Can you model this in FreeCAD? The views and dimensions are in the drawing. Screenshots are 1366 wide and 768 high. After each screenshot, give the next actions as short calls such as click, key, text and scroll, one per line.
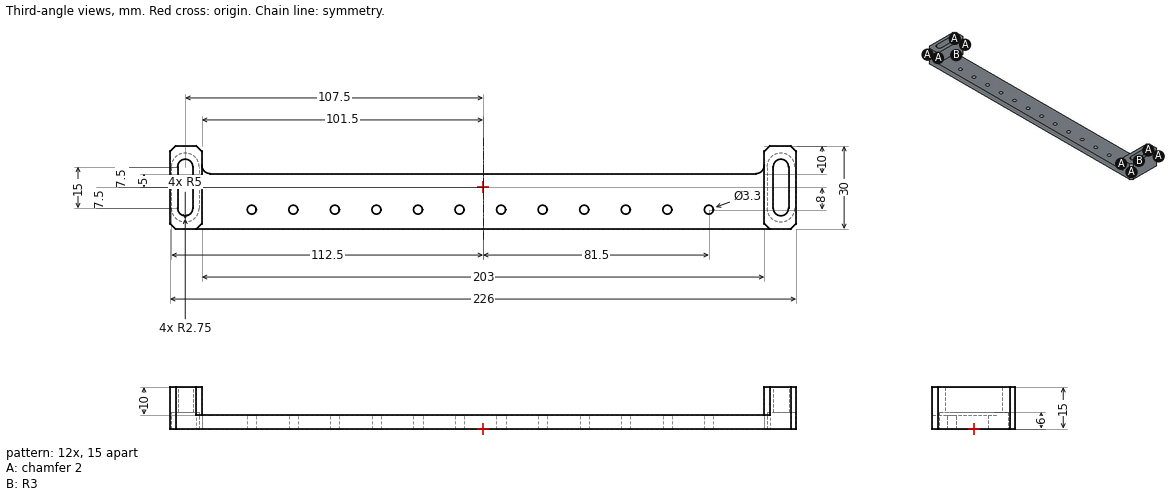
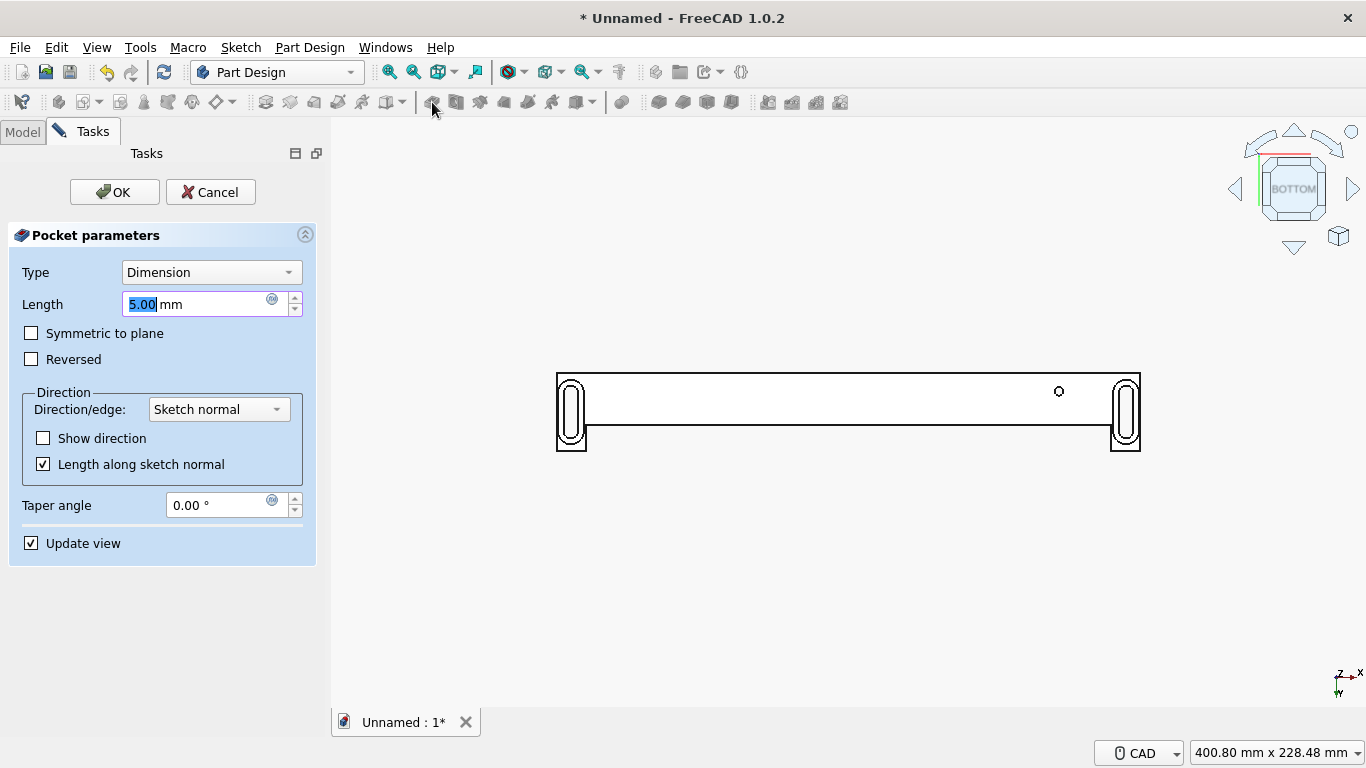
click(212, 272)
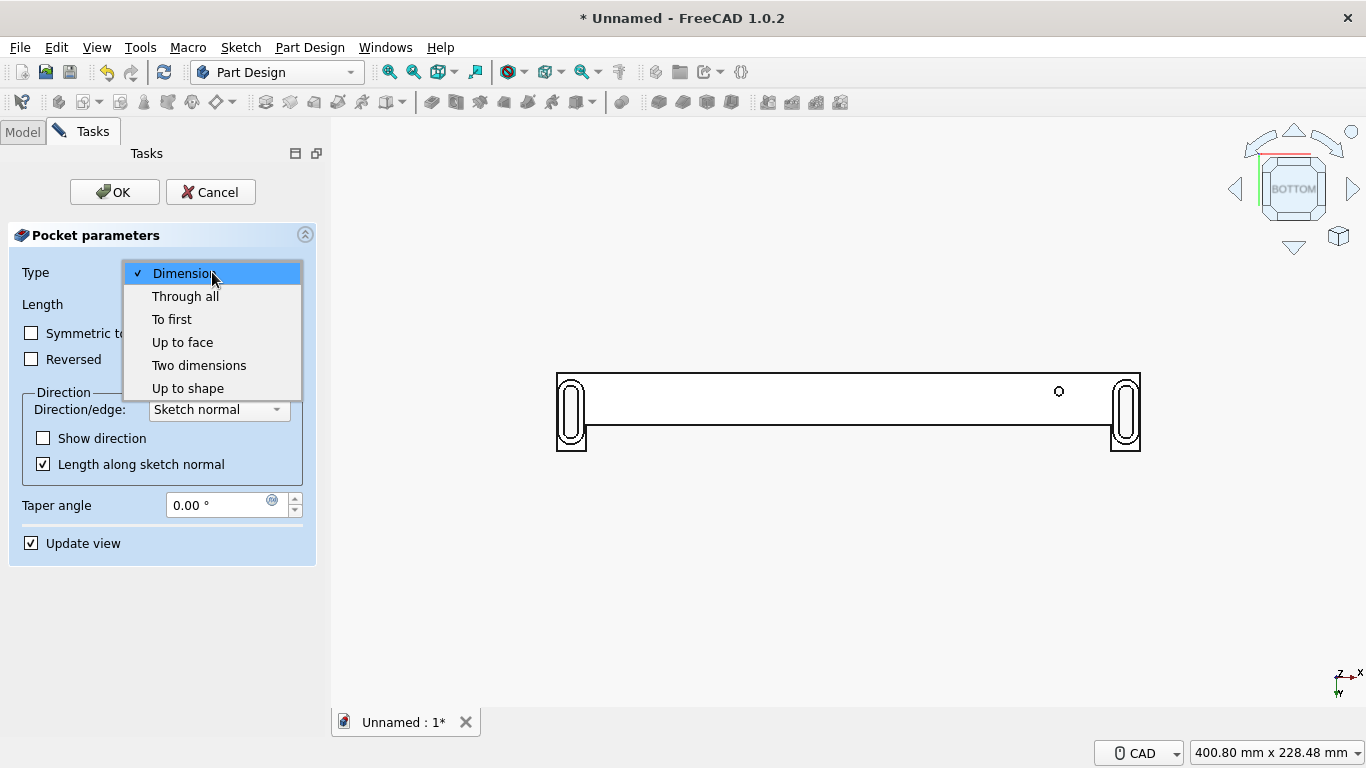
click(212, 296)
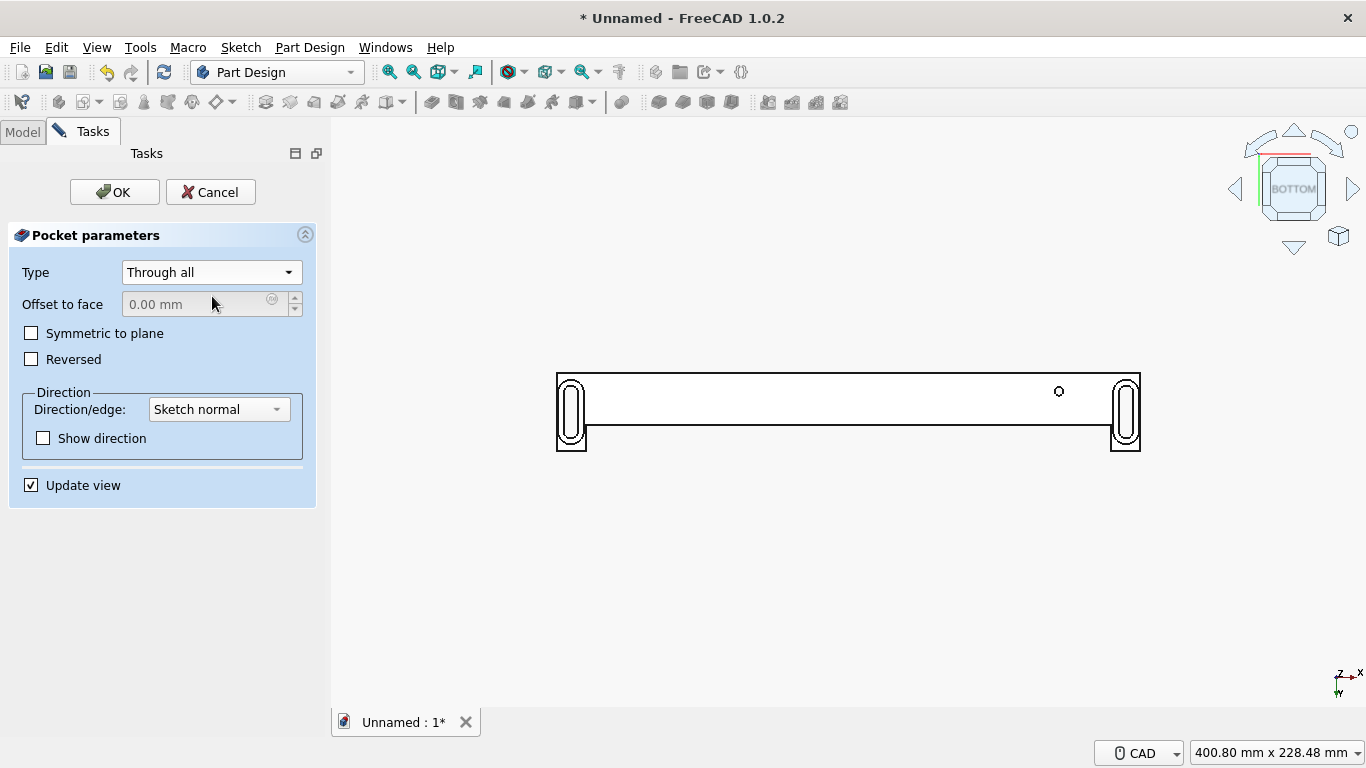
click(115, 192)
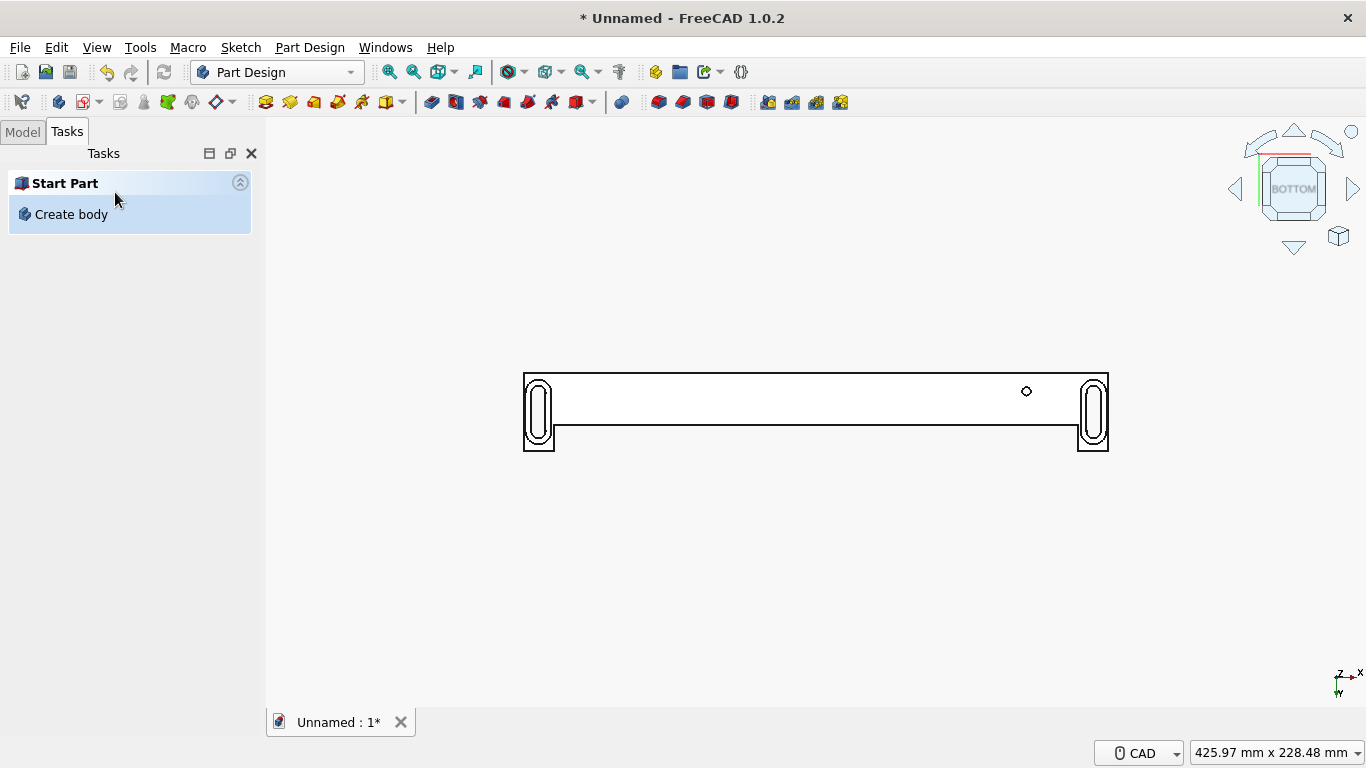
click(23, 131)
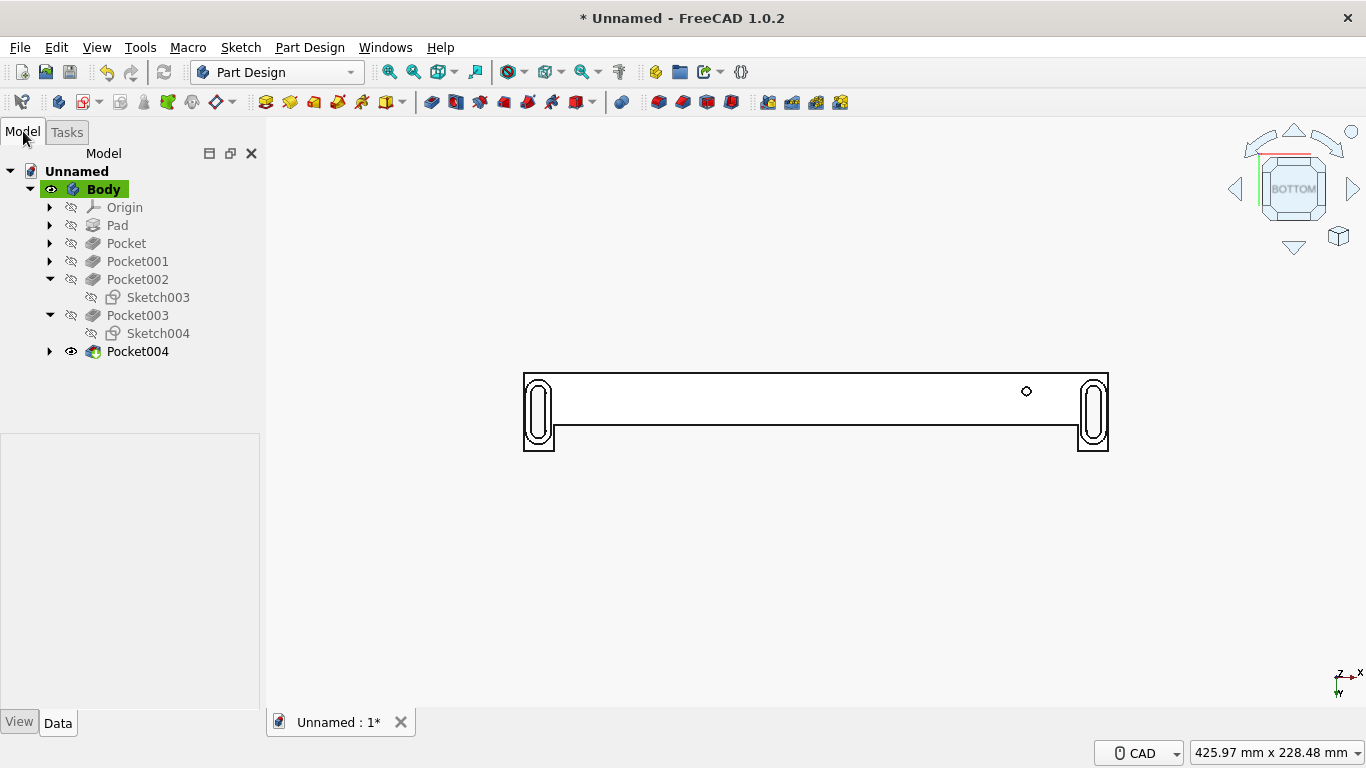
click(116, 351)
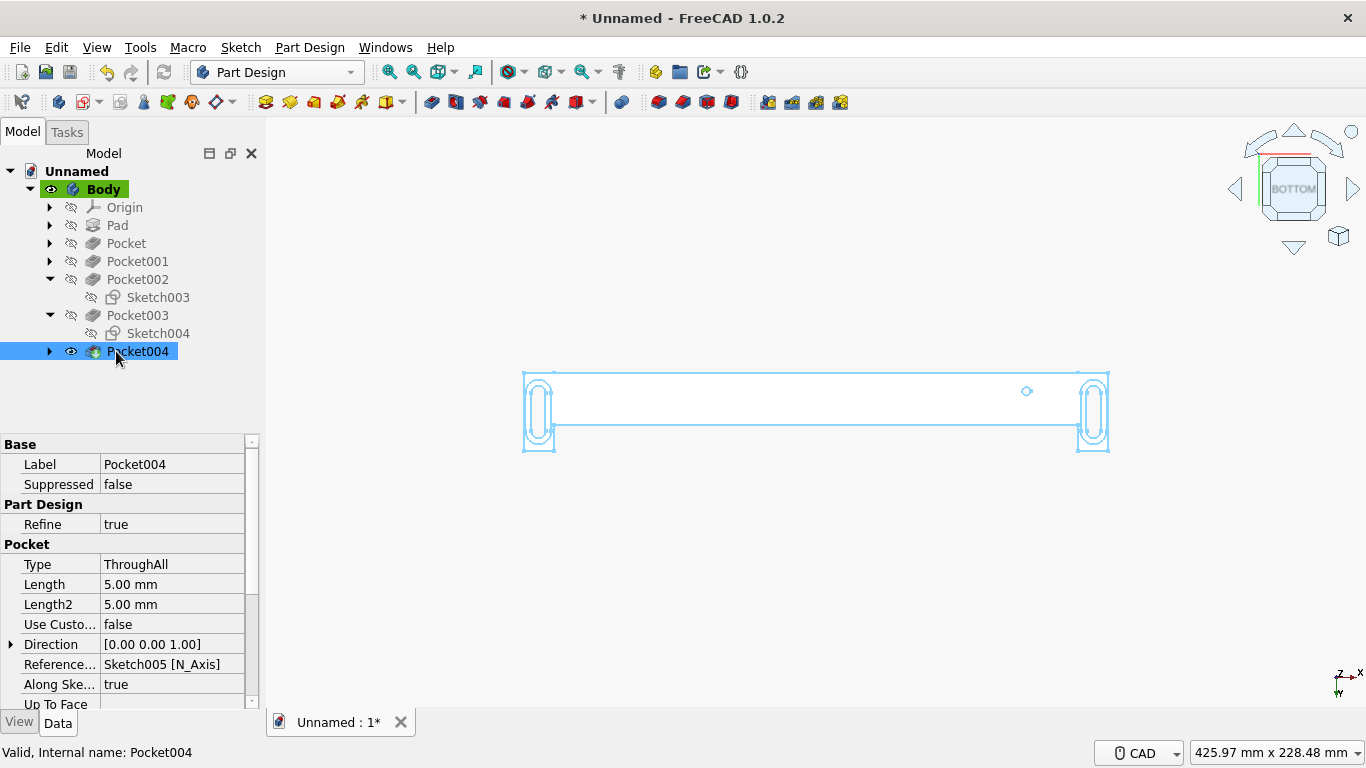
click(792, 102)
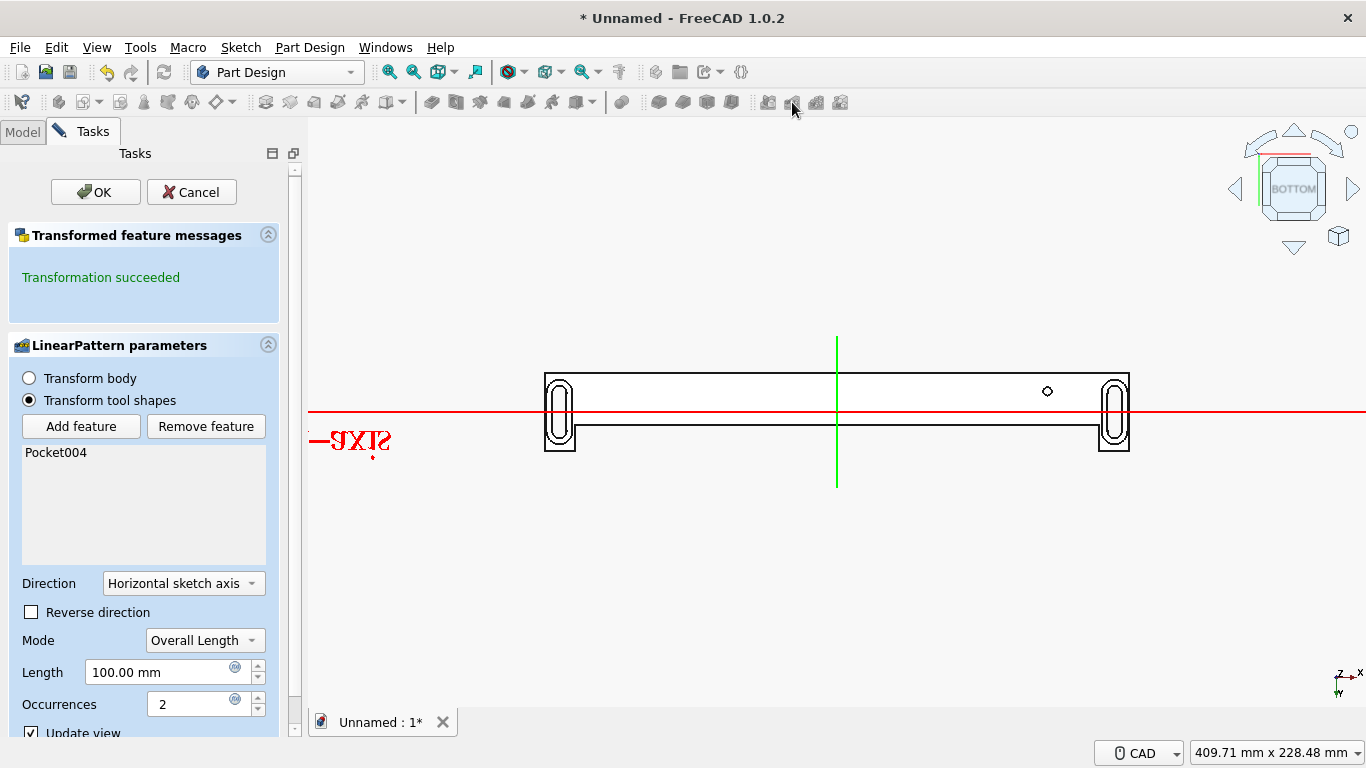
click(184, 584)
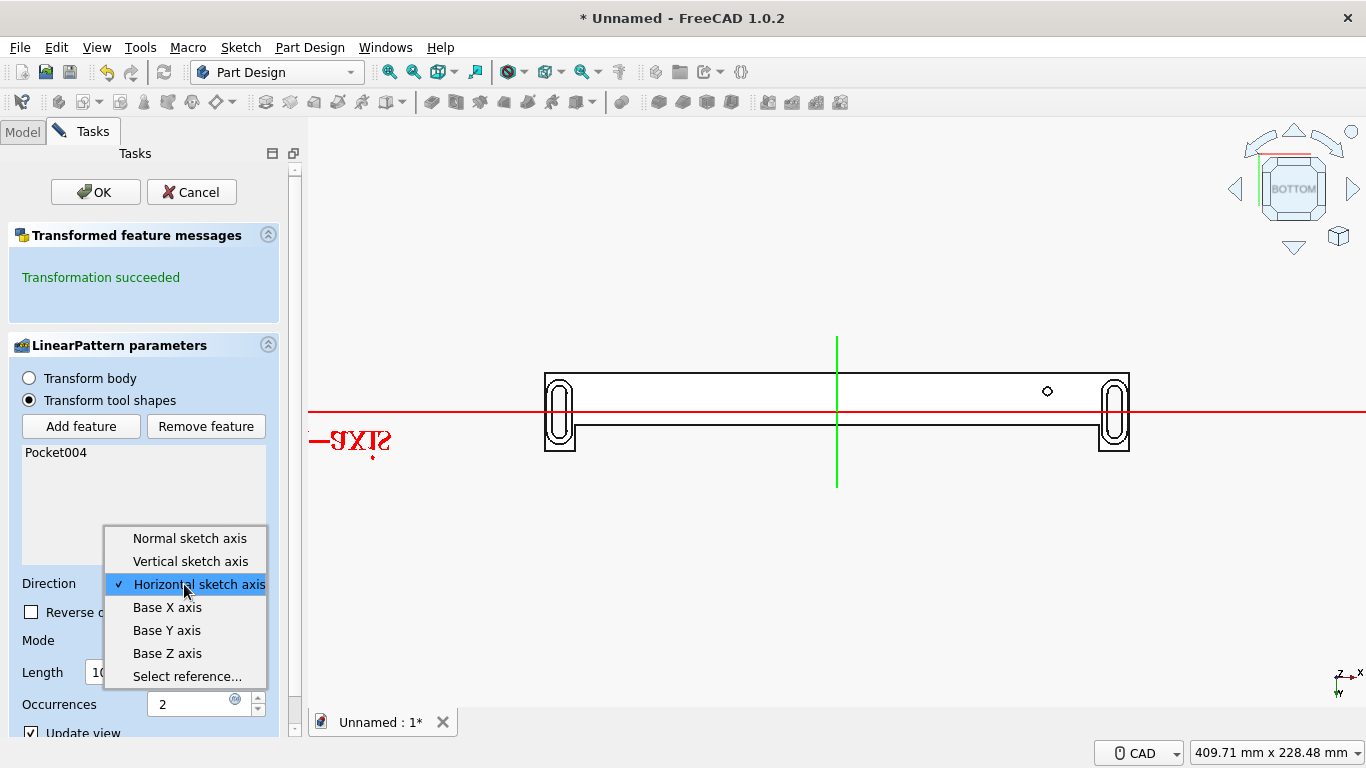
click(184, 608)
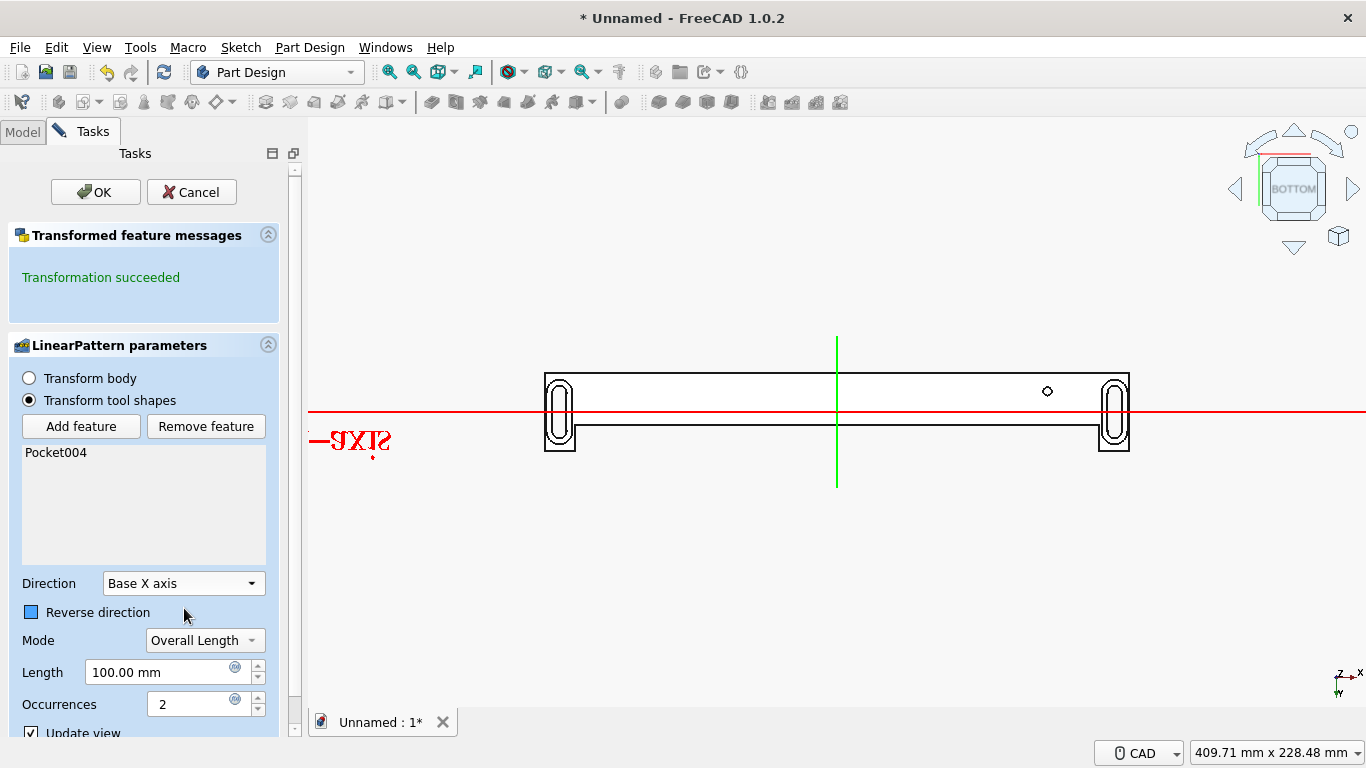
click(206, 640)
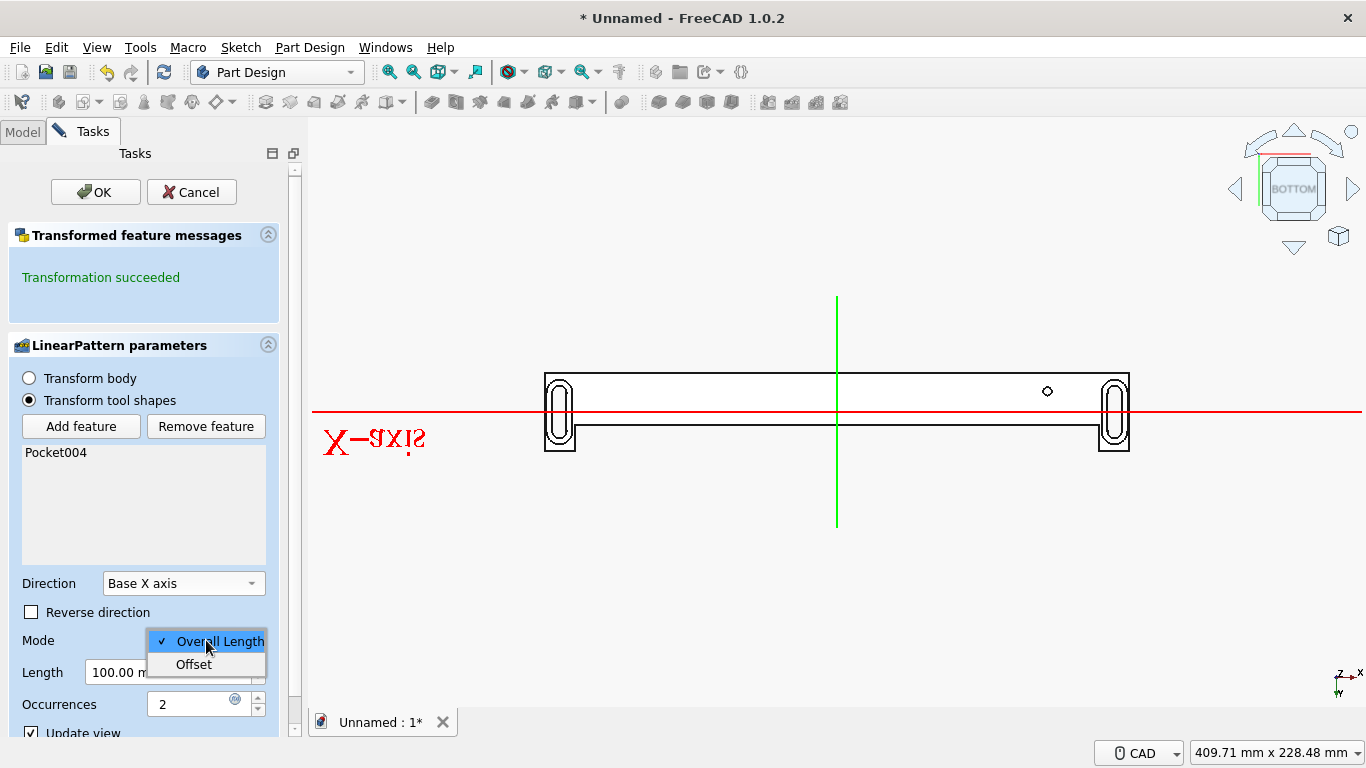
click(206, 664)